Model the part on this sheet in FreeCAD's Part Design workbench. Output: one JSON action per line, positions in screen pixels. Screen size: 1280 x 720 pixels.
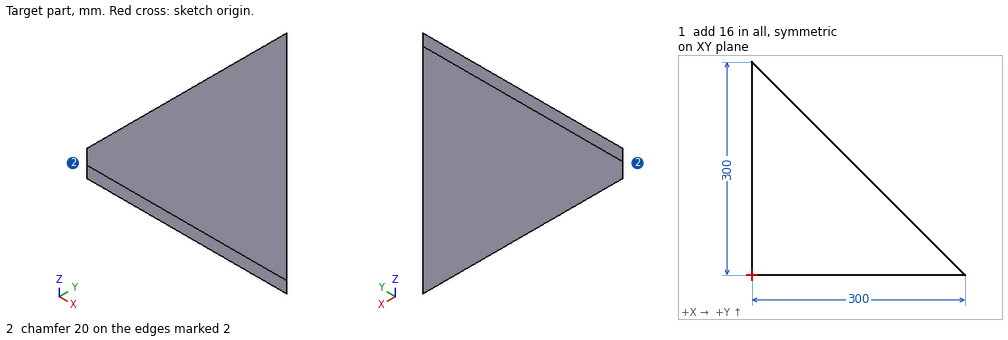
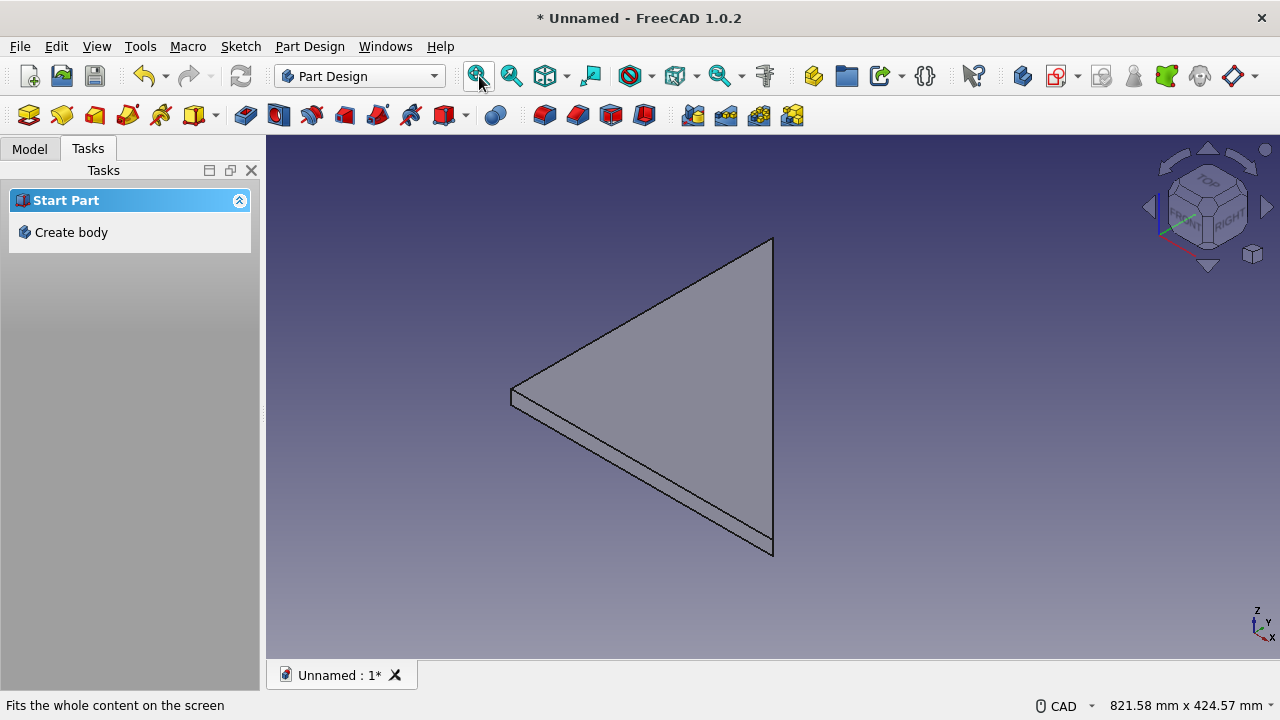
{"action": "scroll", "coordinate": [511, 396], "scroll_direction": "up", "scroll_amount": 4}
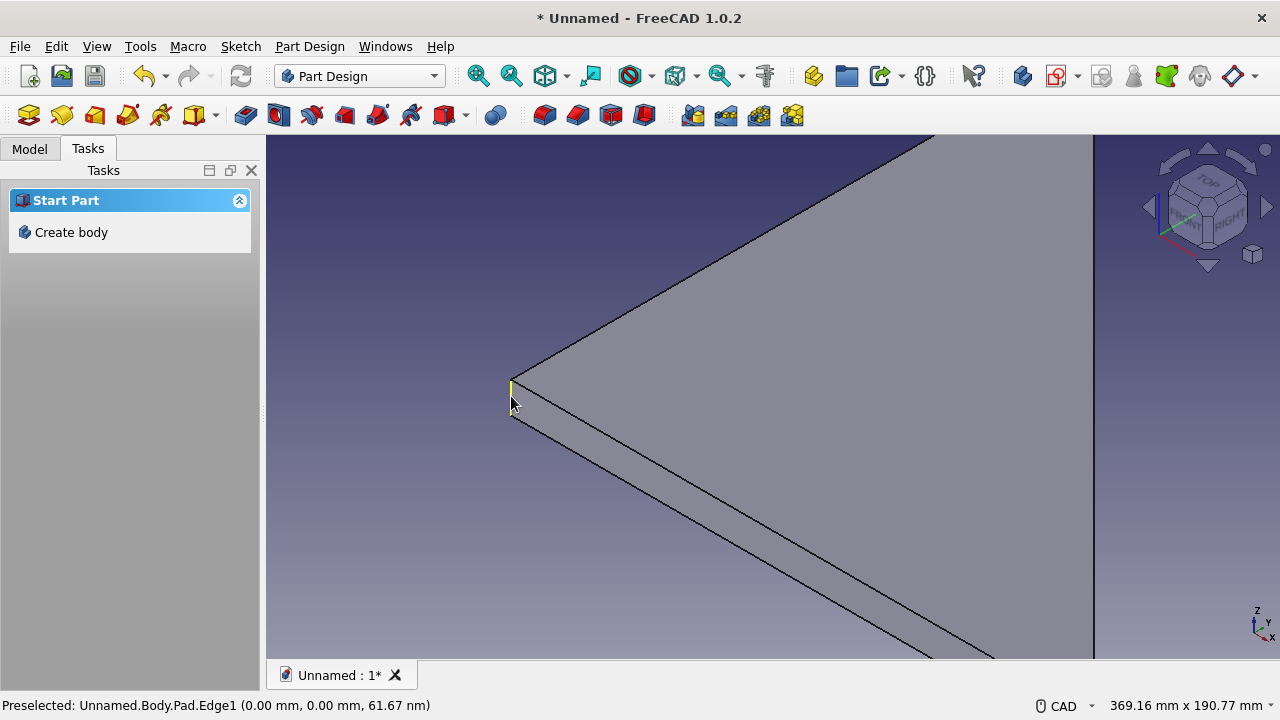
{"action": "left_click", "coordinate": [479, 76]}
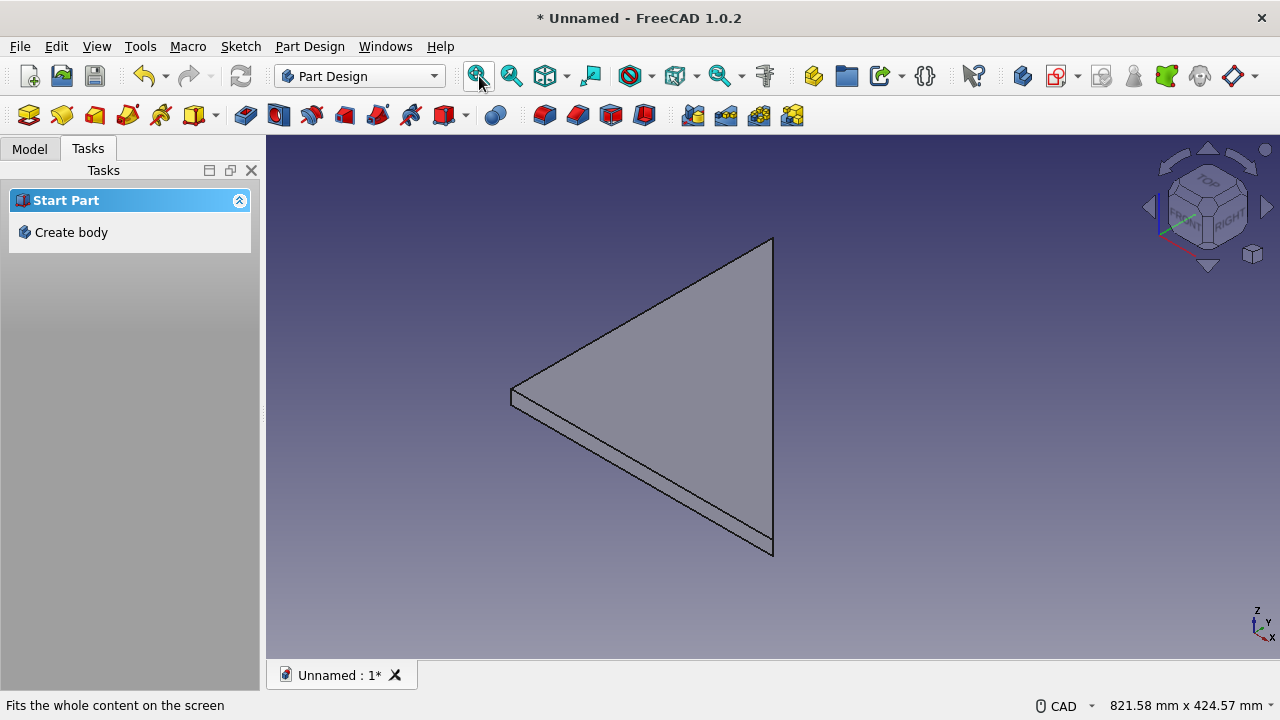
{"action": "key", "text": "2"}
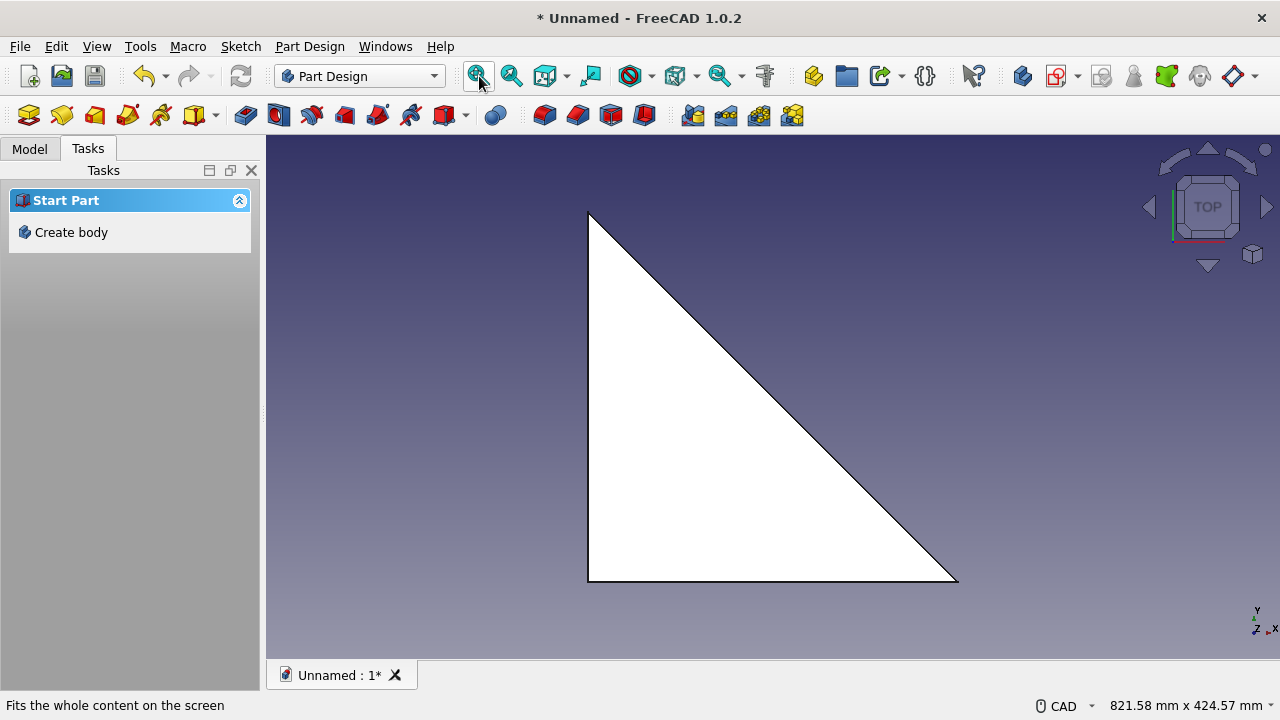
{"action": "scroll", "coordinate": [588, 581], "scroll_direction": "up", "scroll_amount": 4}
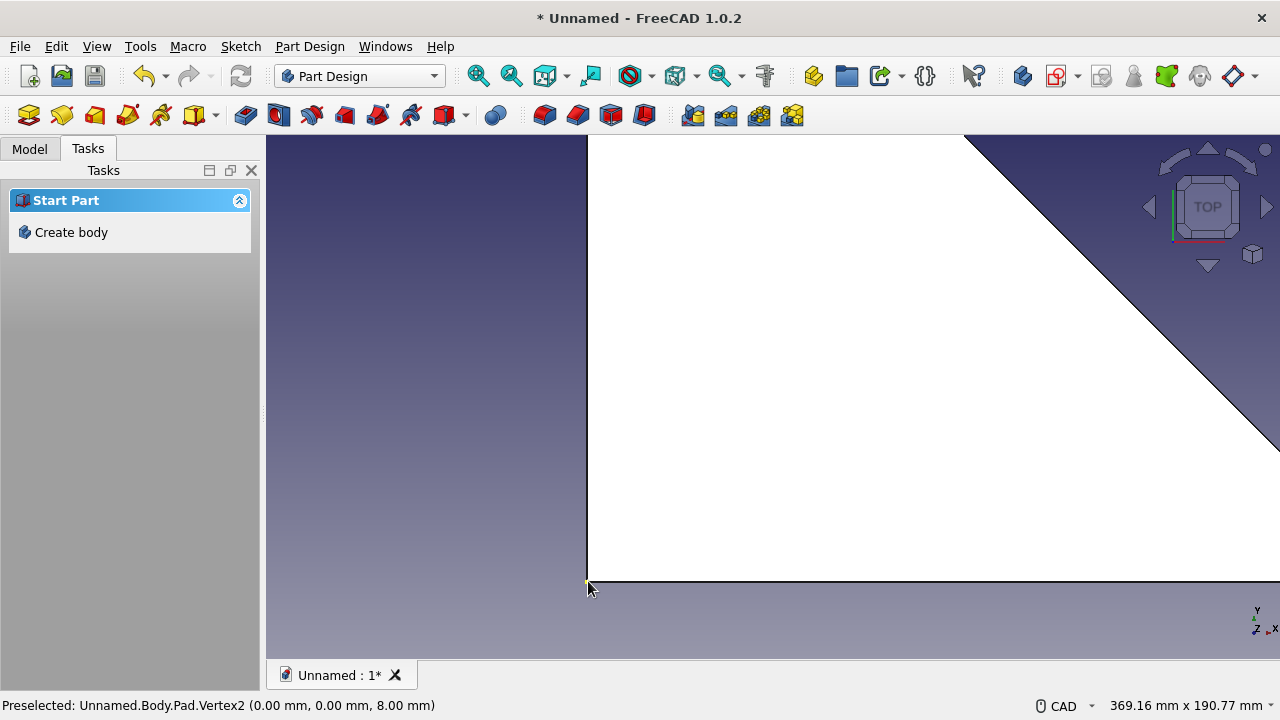
{"action": "left_click", "coordinate": [479, 76]}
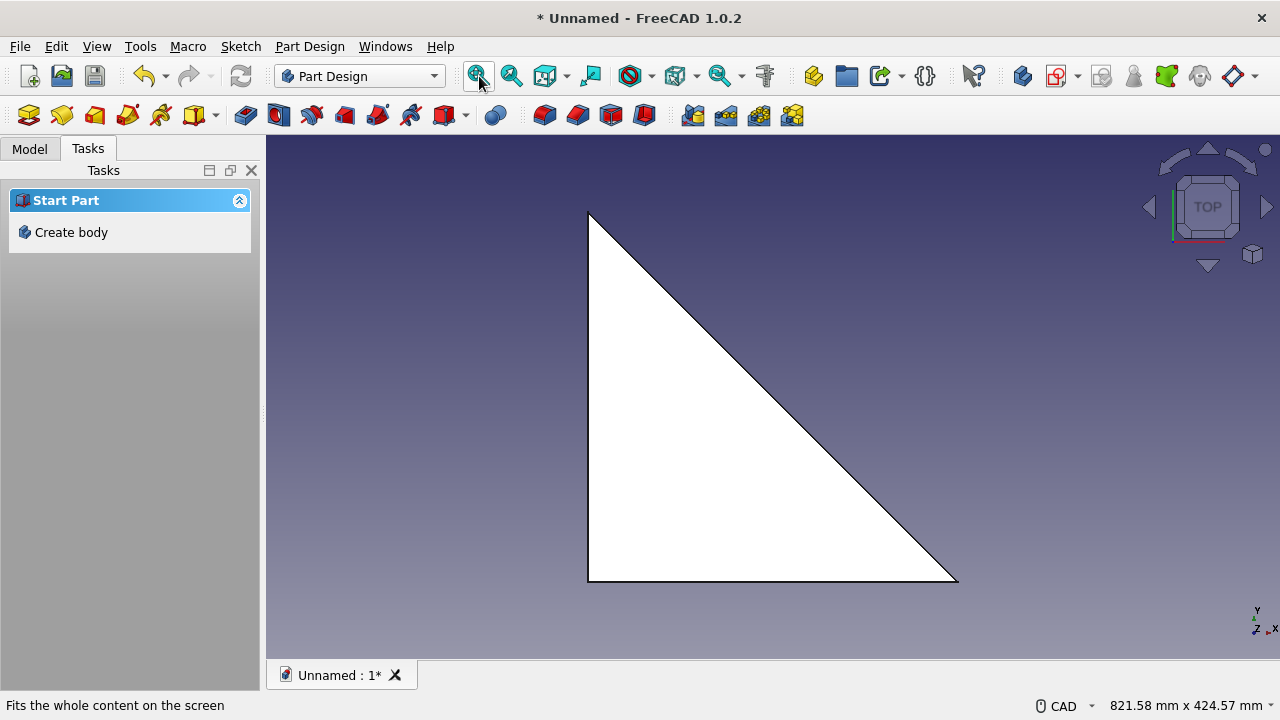
{"action": "key", "text": "1"}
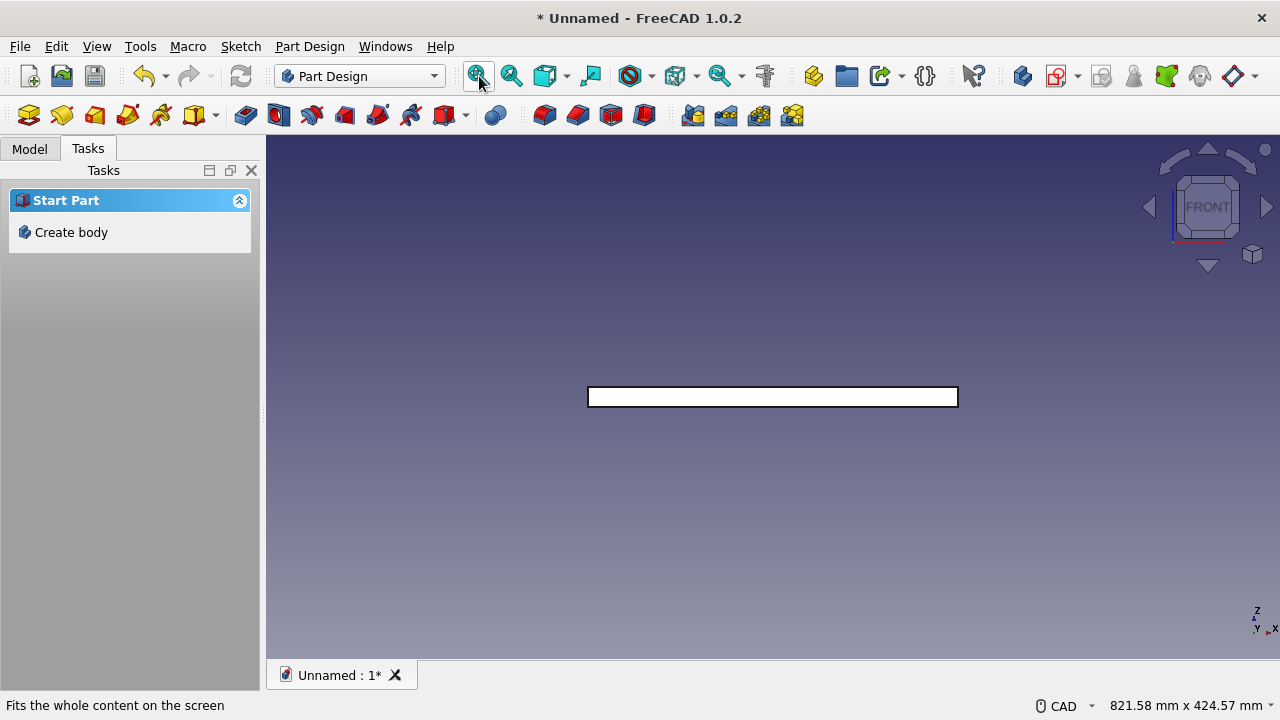
{"action": "left_click", "coordinate": [479, 76]}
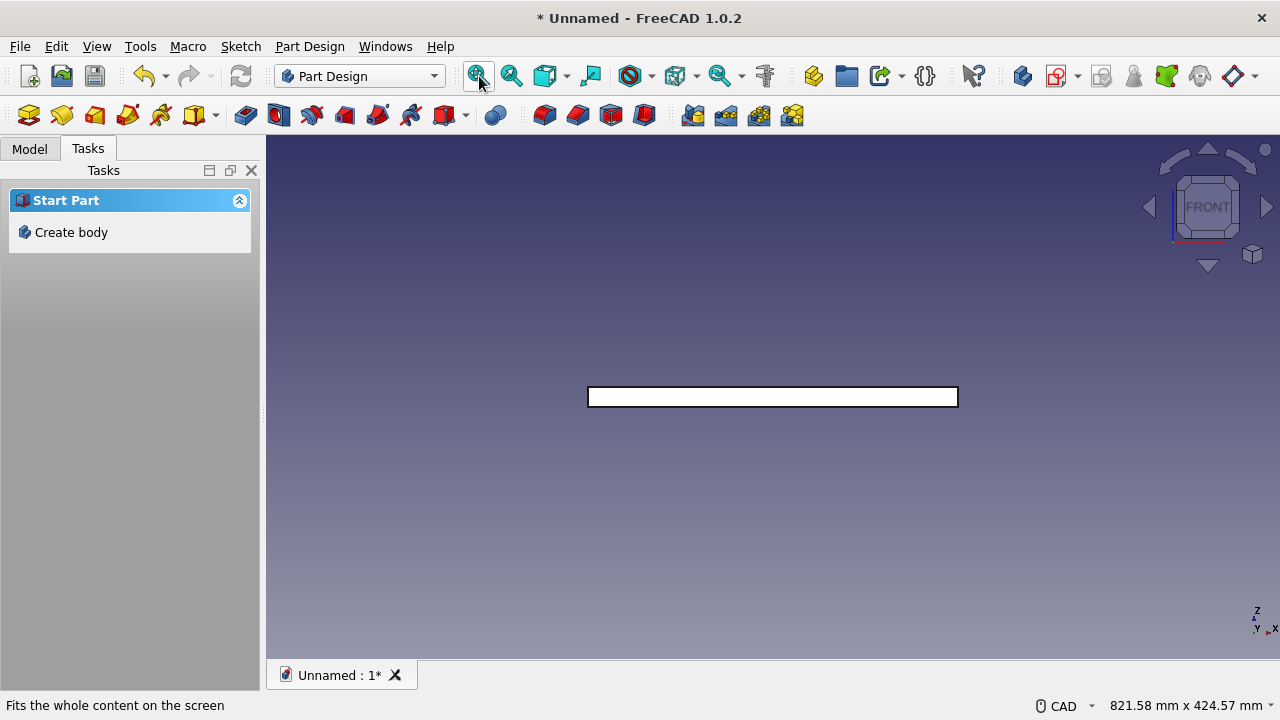
{"action": "left_click", "coordinate": [588, 396]}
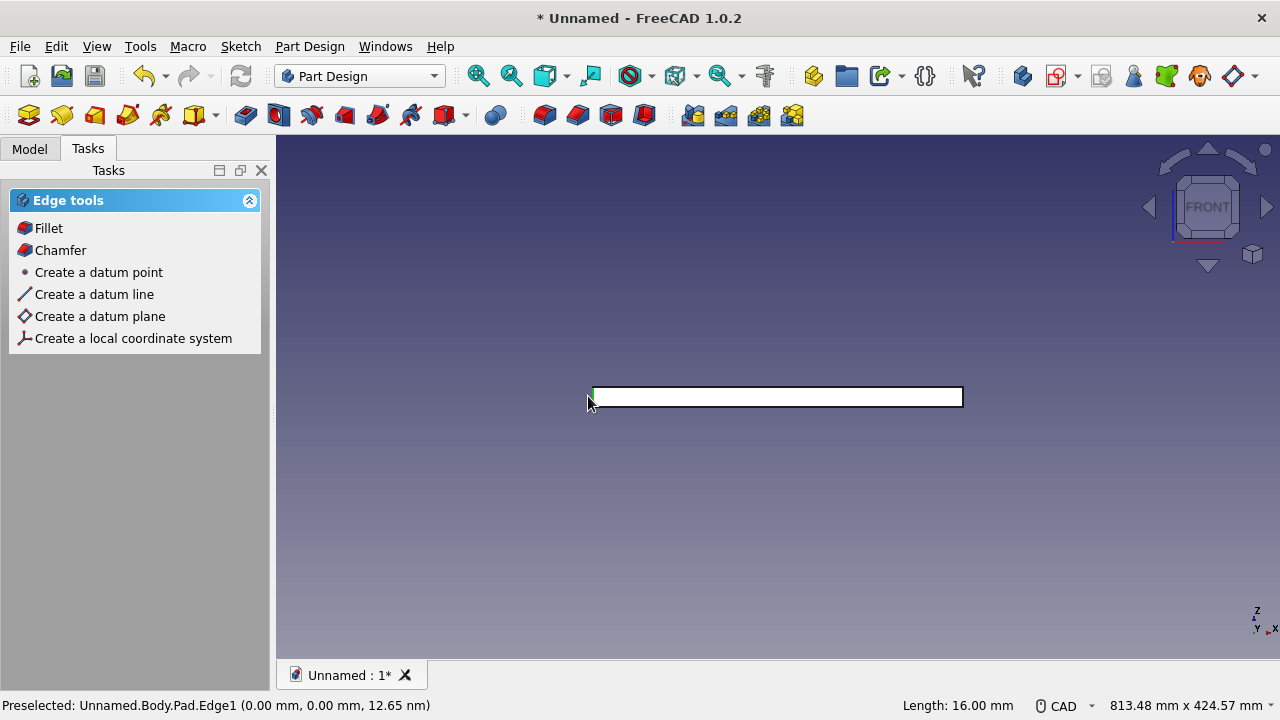
{"action": "left_click", "coordinate": [578, 116]}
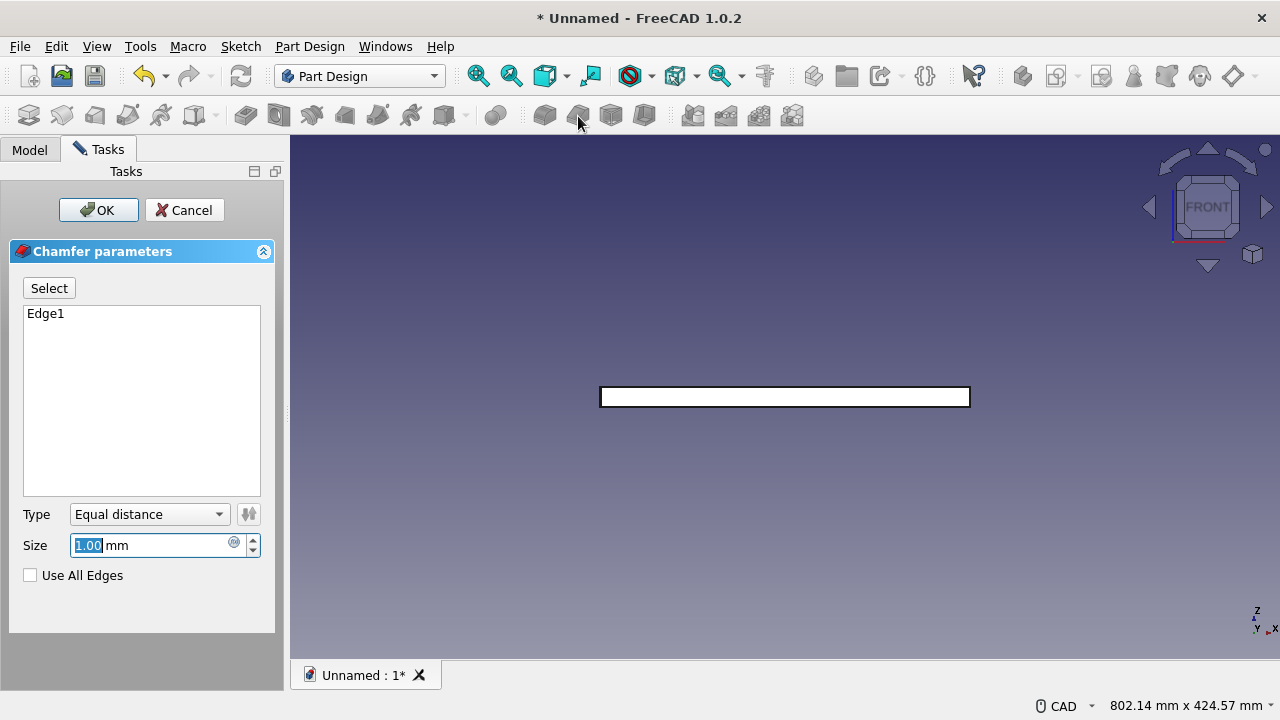
{"action": "type", "text": "20"}
{"action": "key", "text": "Tab"}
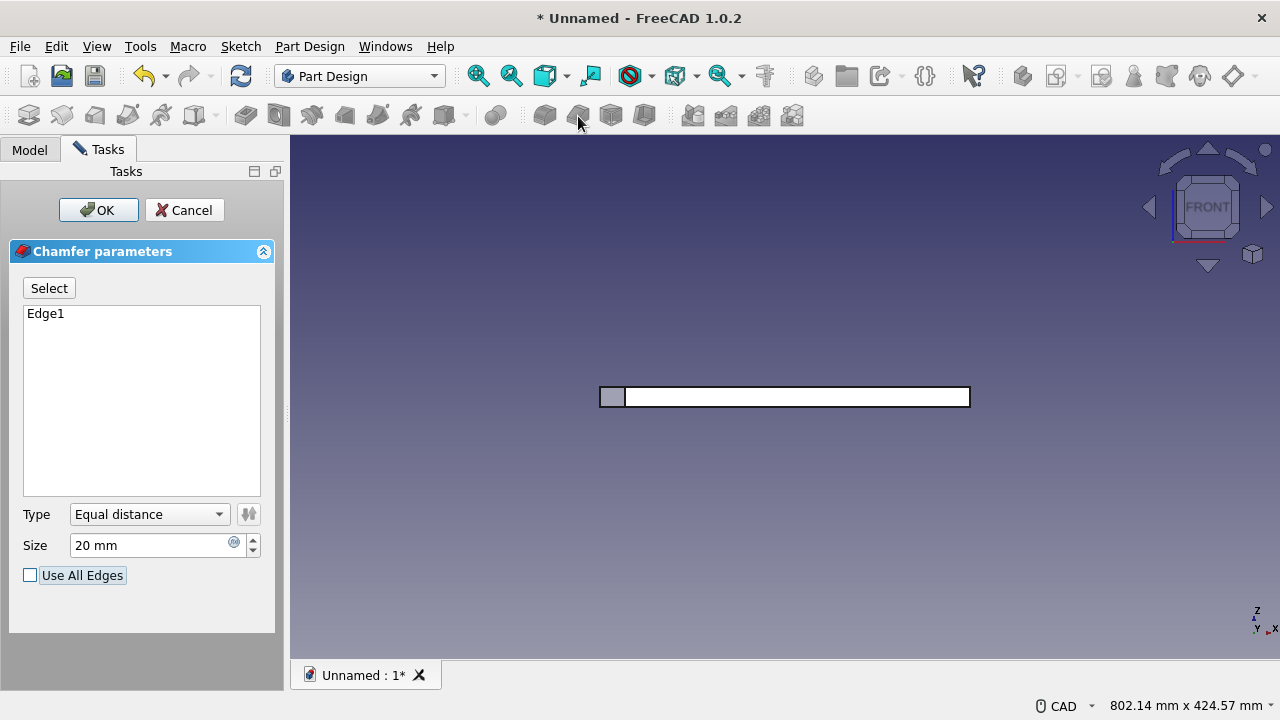
{"action": "left_click", "coordinate": [99, 210]}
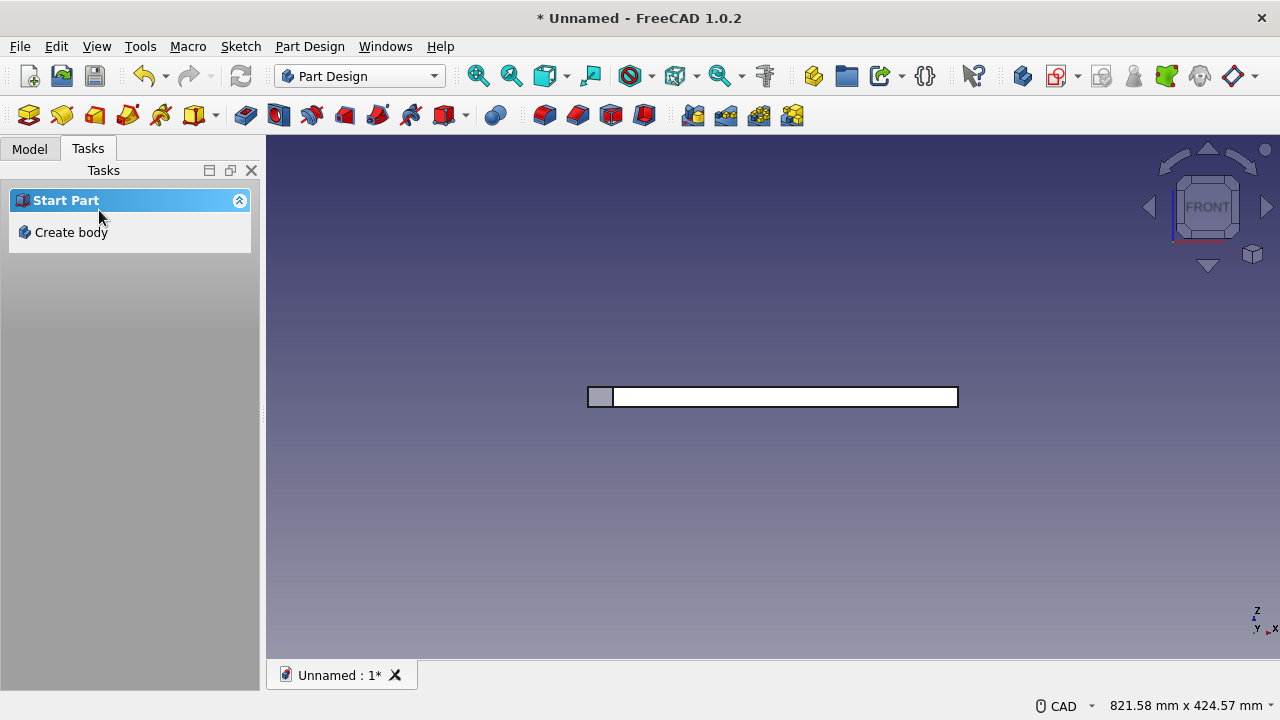
{"action": "key", "text": "0"}